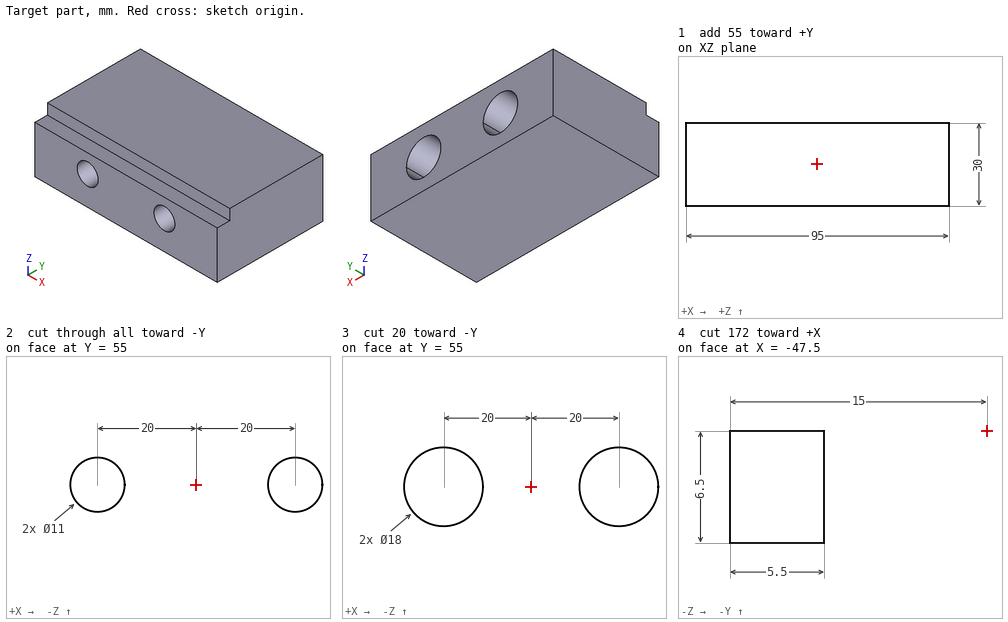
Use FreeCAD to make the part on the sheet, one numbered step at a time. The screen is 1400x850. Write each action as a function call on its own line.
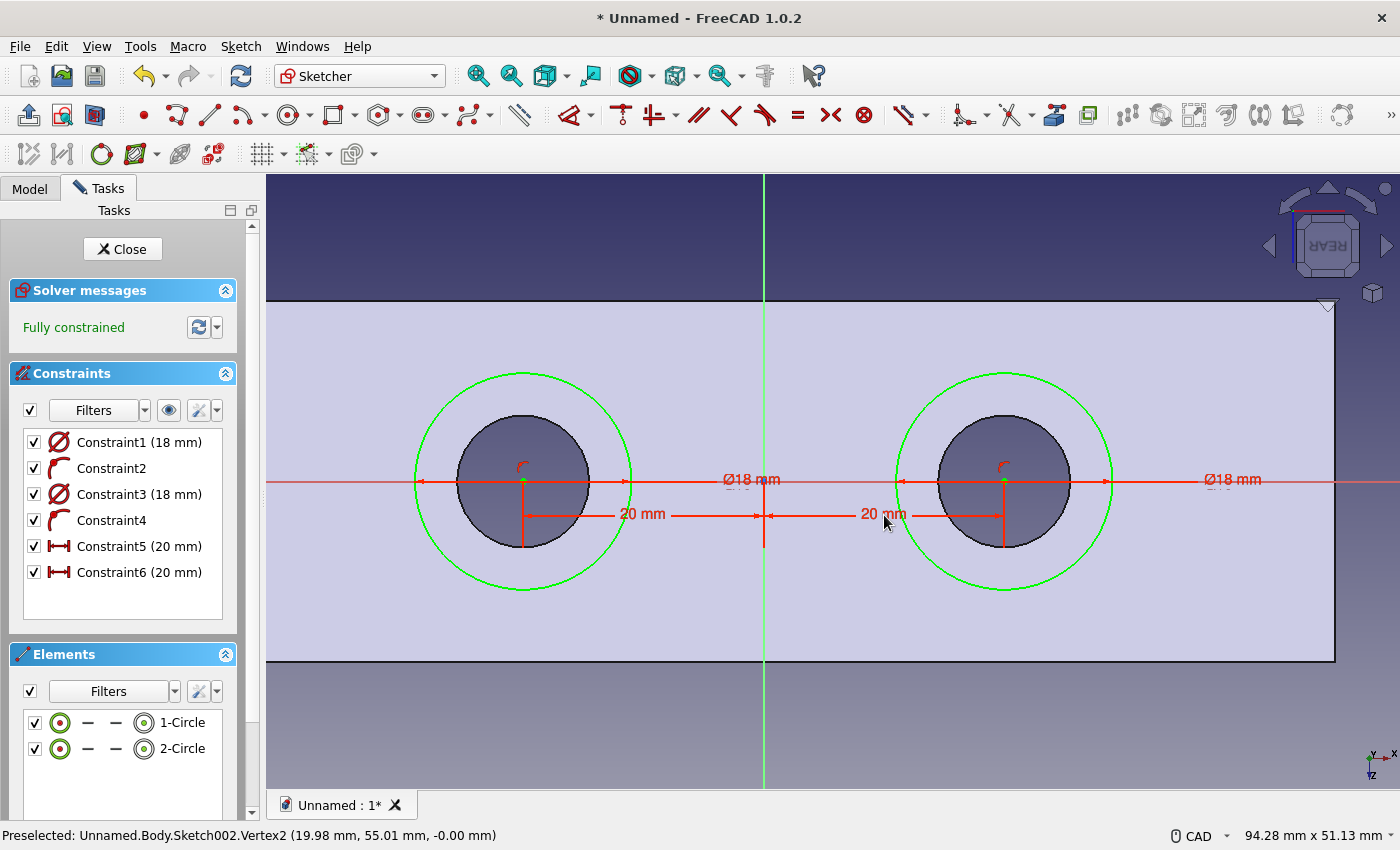
click(123, 249)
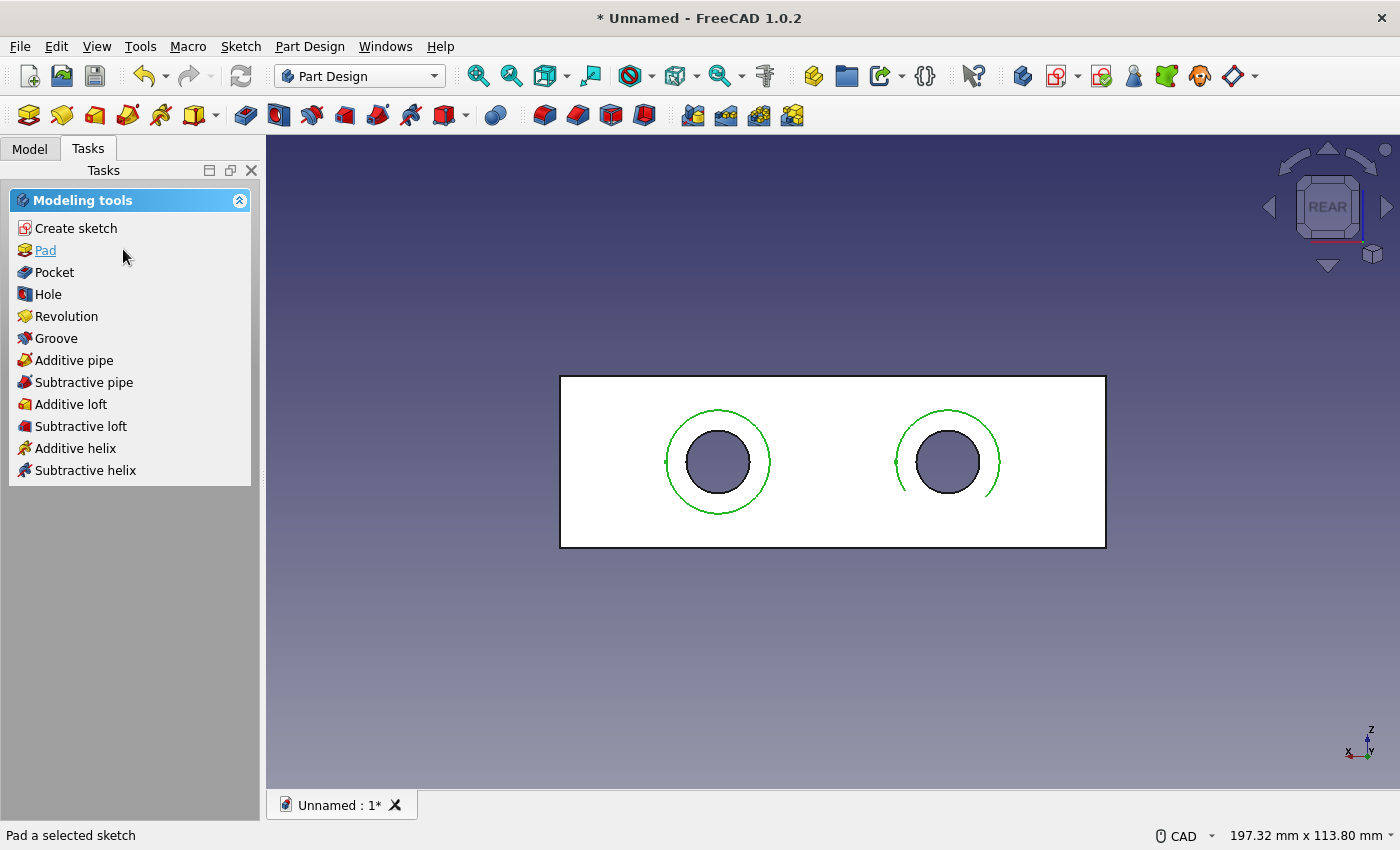
click(246, 116)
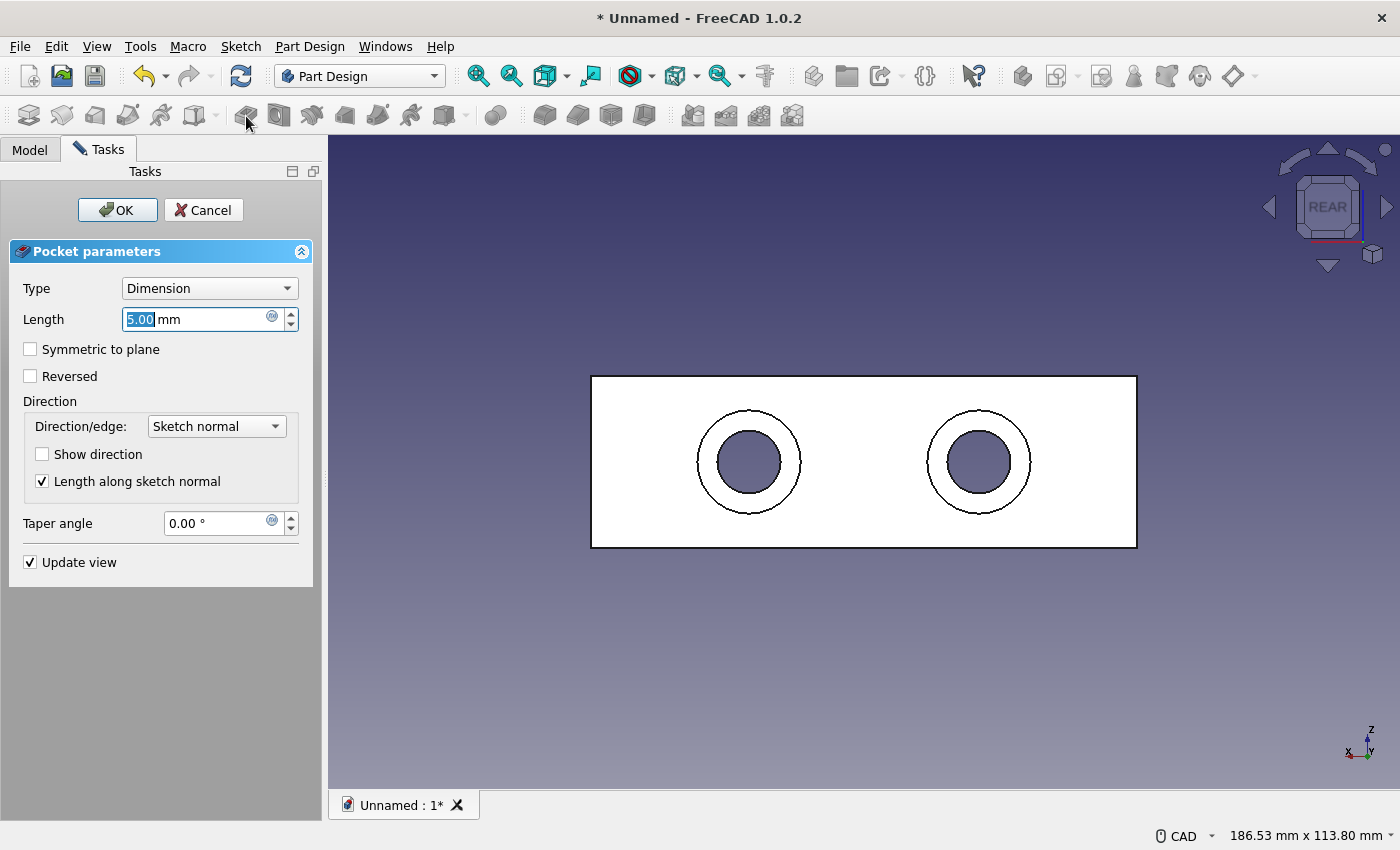
text(20)
key(Tab)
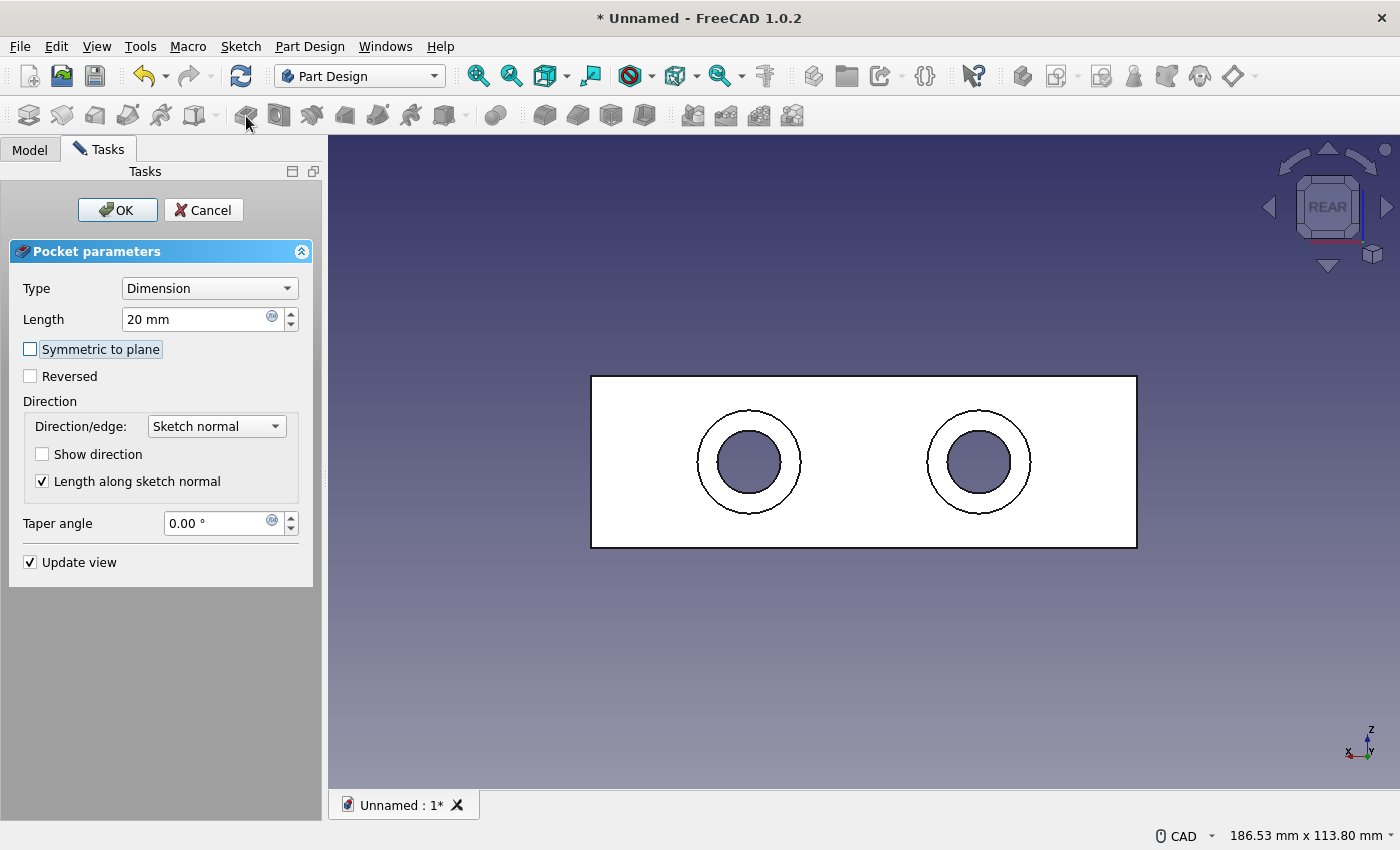
click(118, 210)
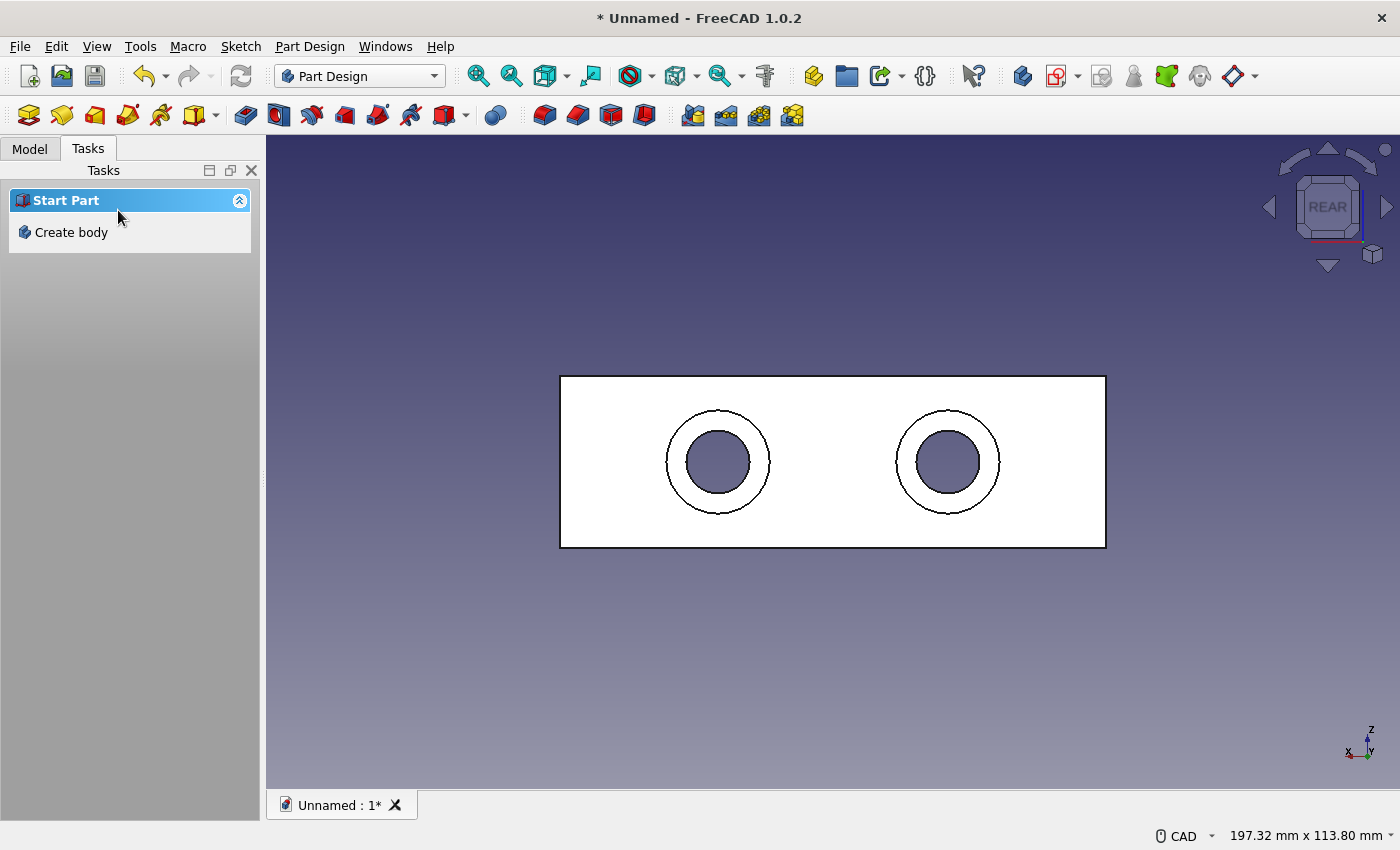
key(6)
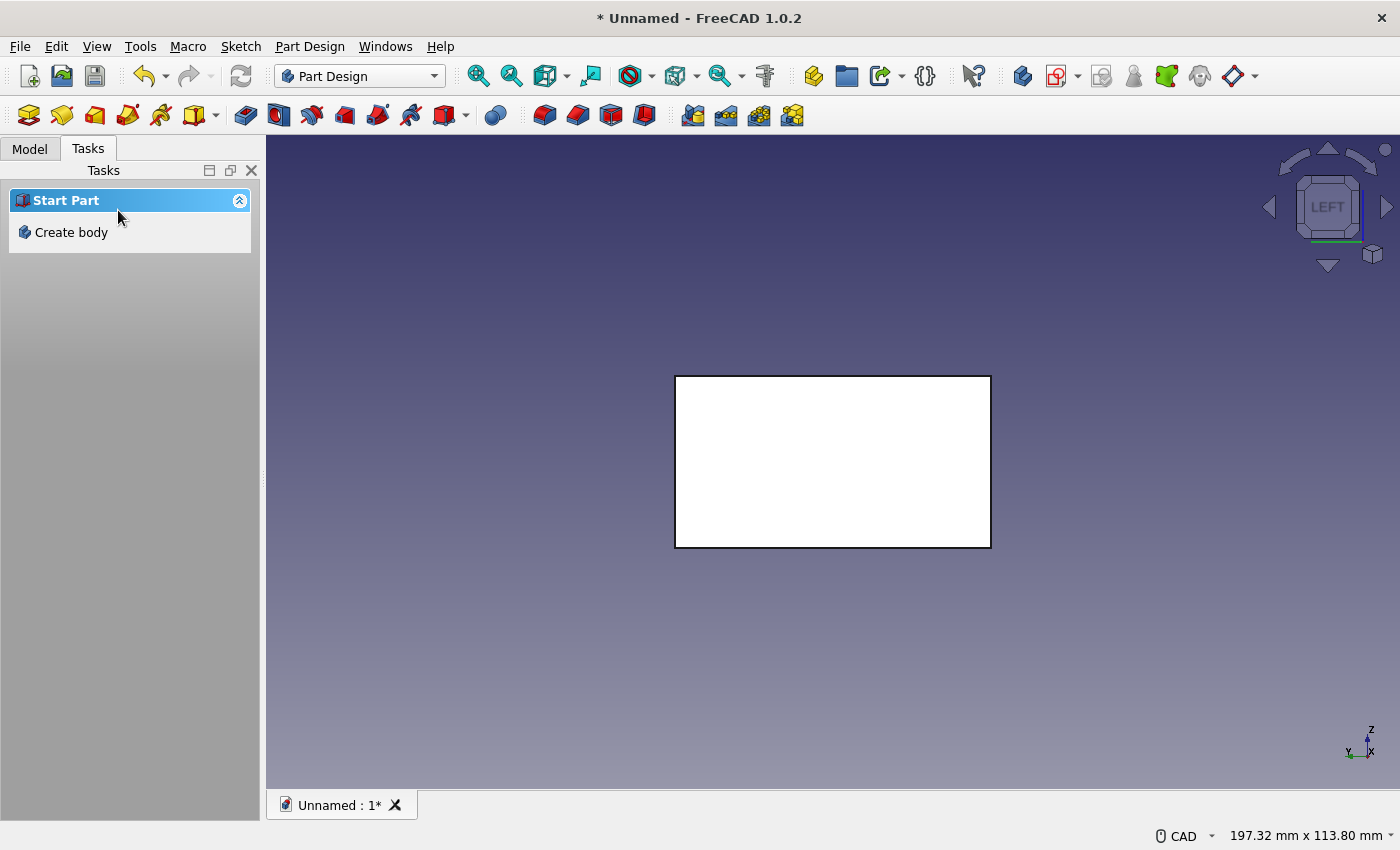
click(479, 76)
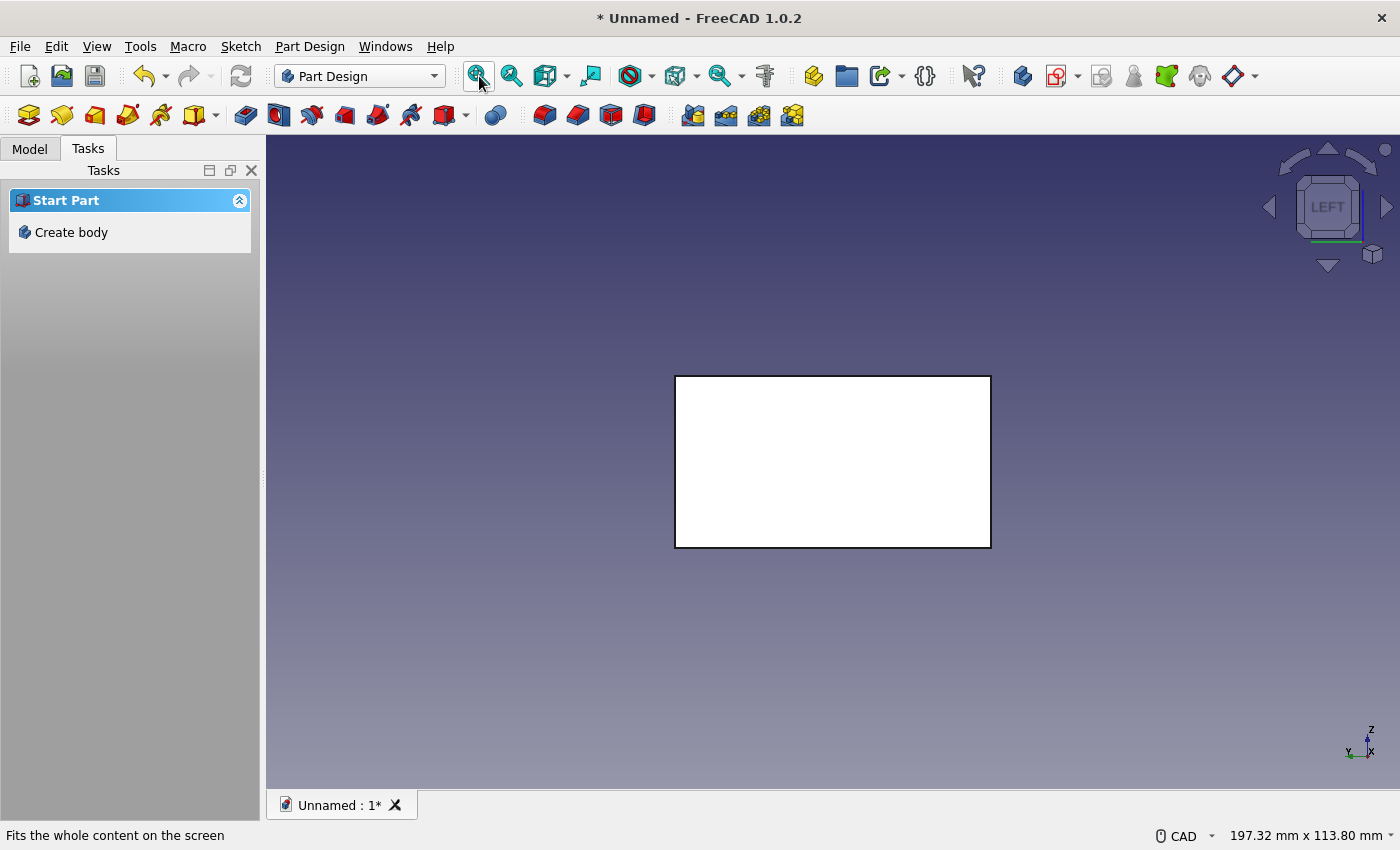
click(788, 461)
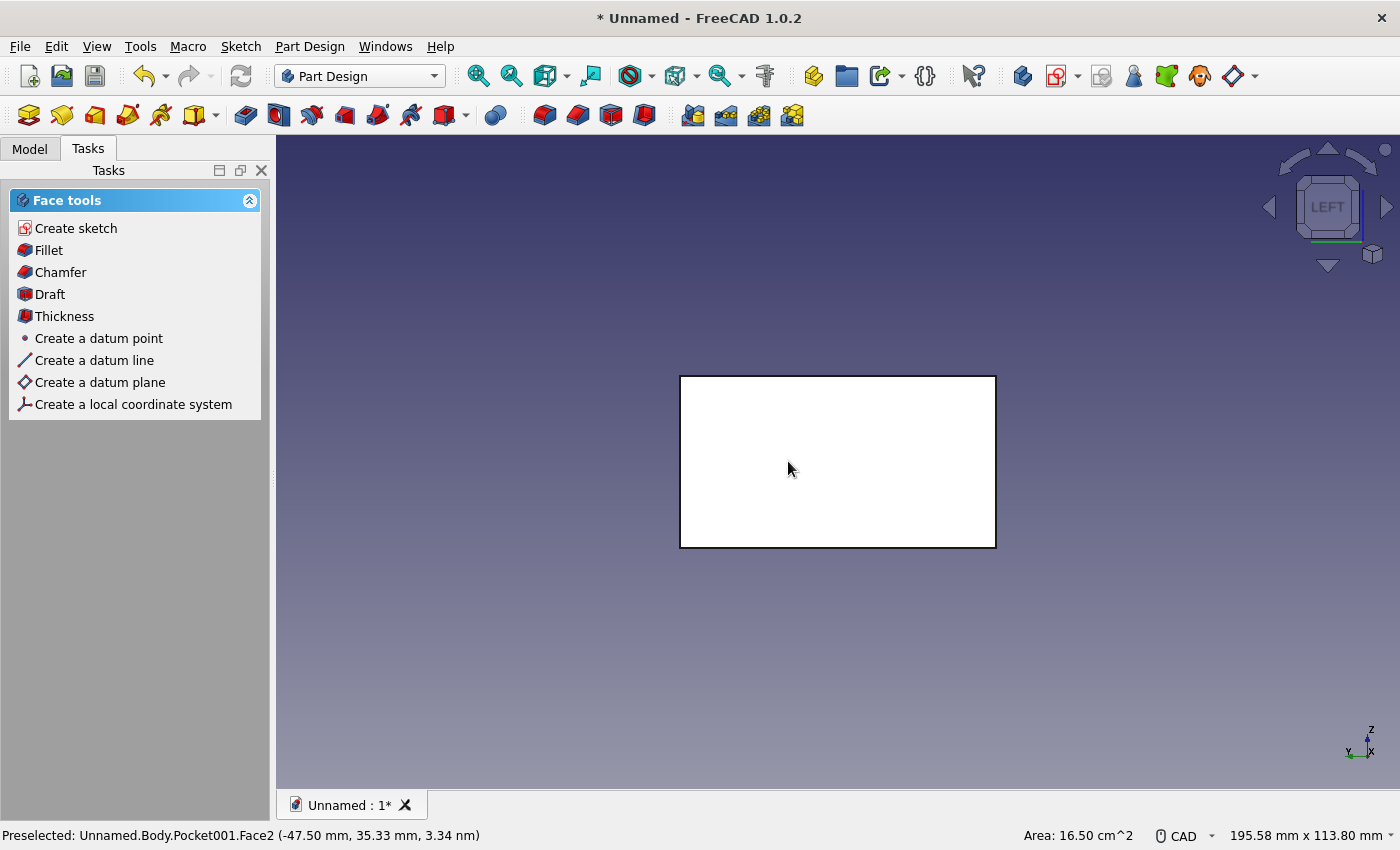
click(1056, 76)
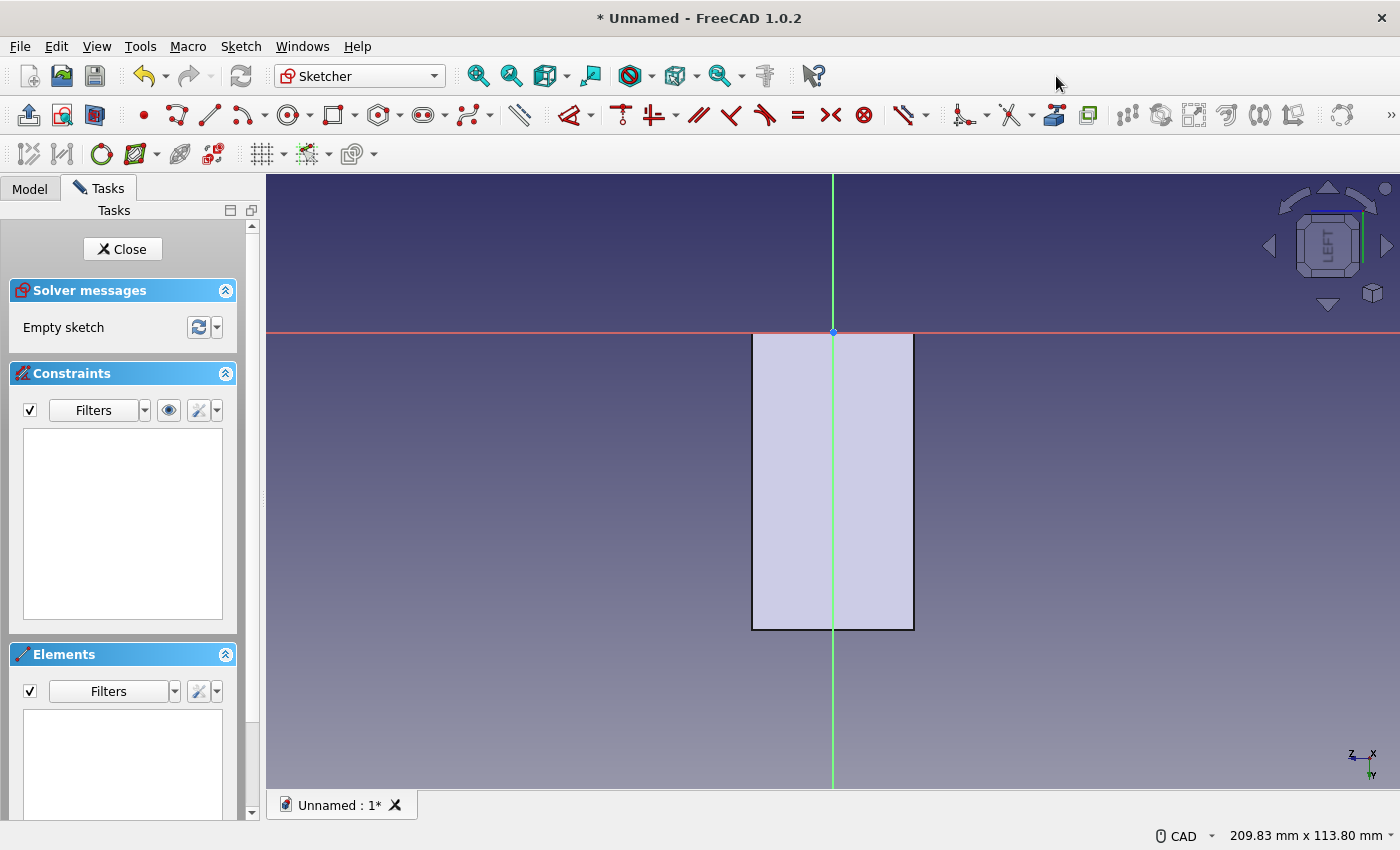
scroll(796, 334, up, 11)